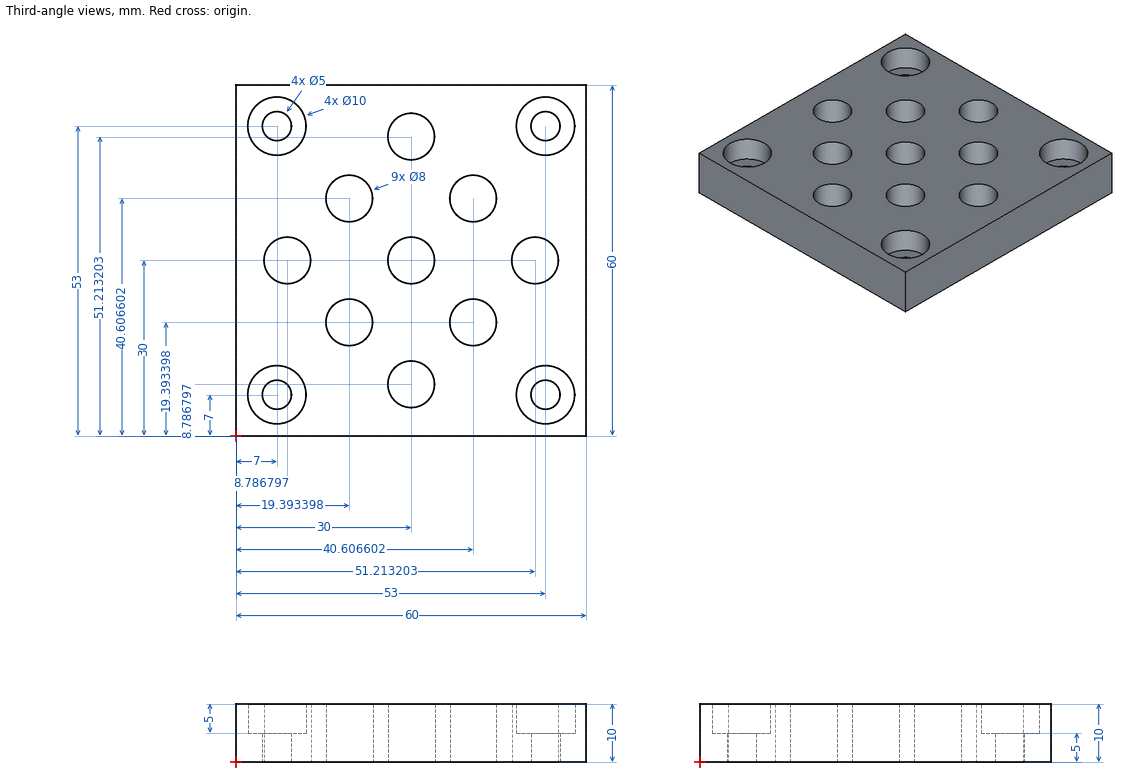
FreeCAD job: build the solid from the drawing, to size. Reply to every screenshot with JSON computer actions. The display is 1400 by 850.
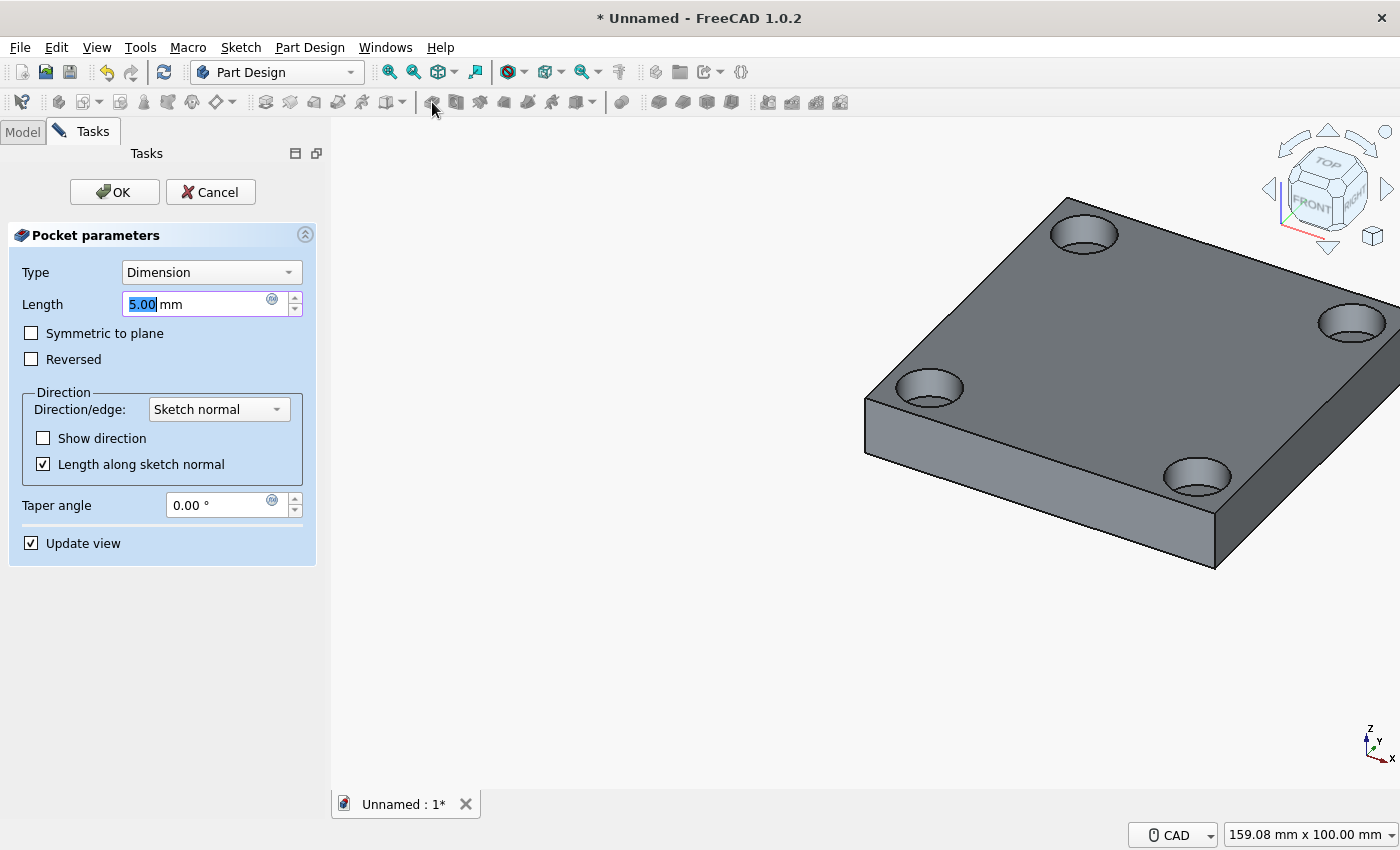
{"action": "type", "text": "5"}
{"action": "key", "text": "Tab"}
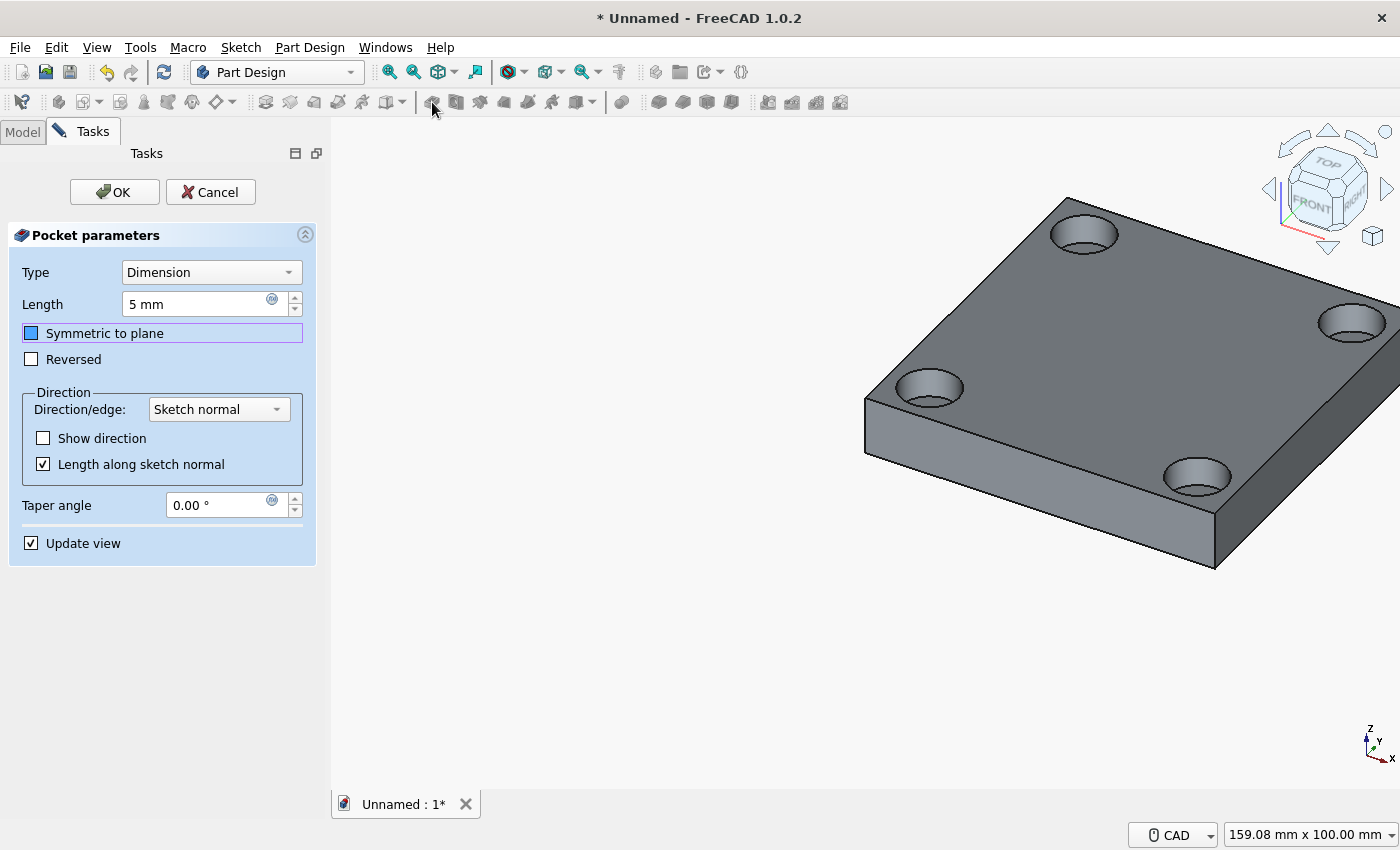
{"action": "left_click", "coordinate": [115, 192]}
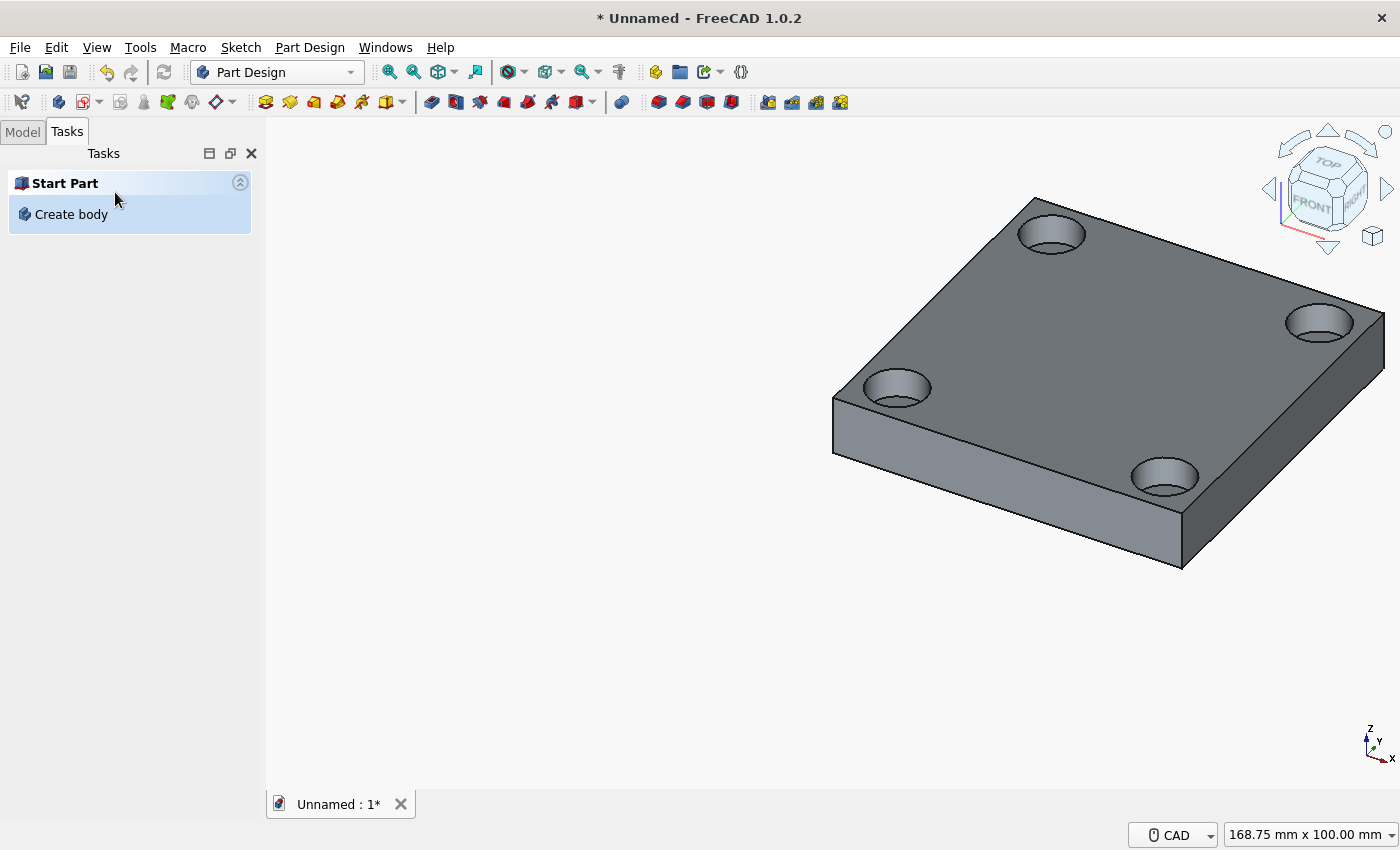
{"action": "key", "text": "0"}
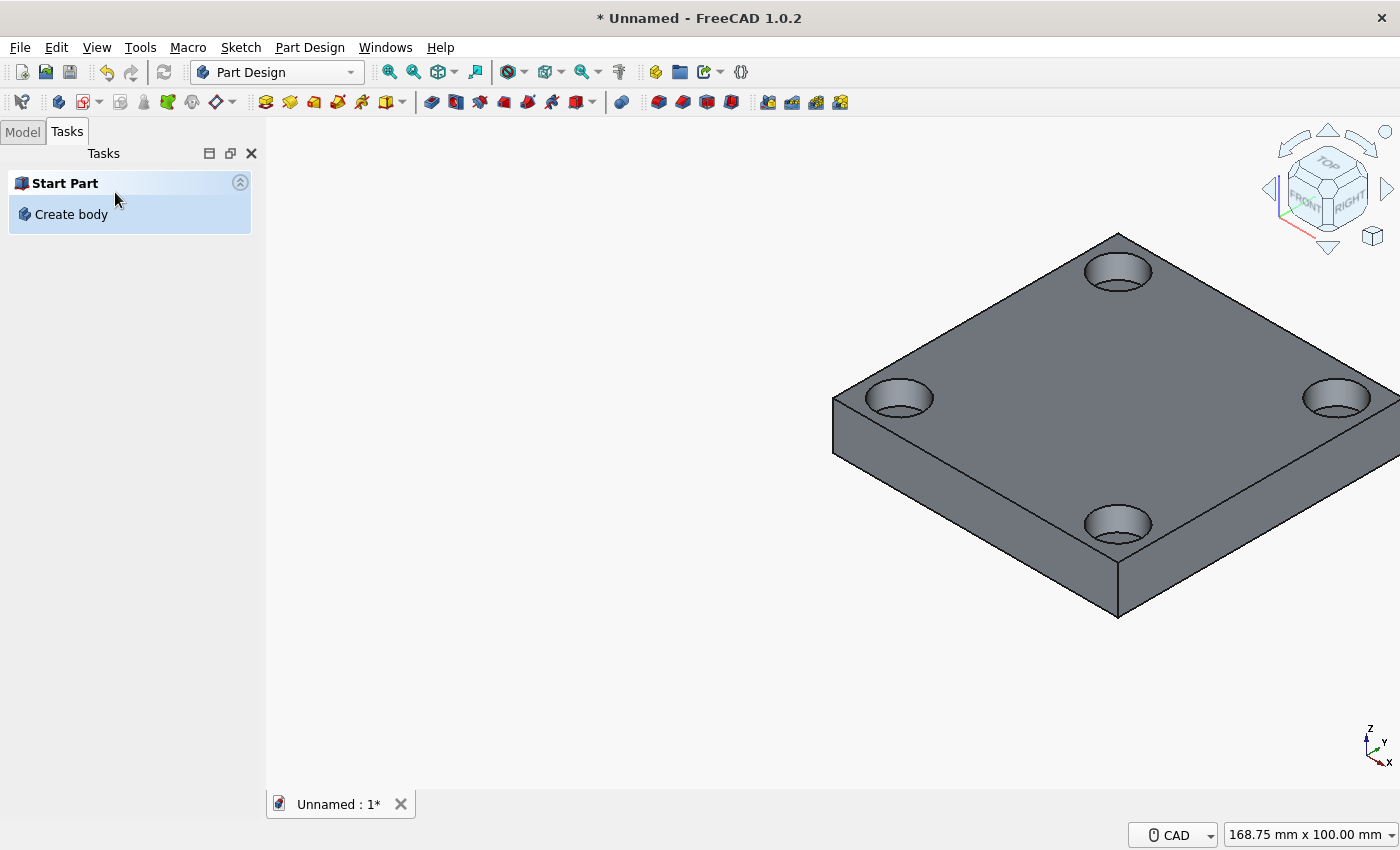
{"action": "left_click", "coordinate": [390, 72]}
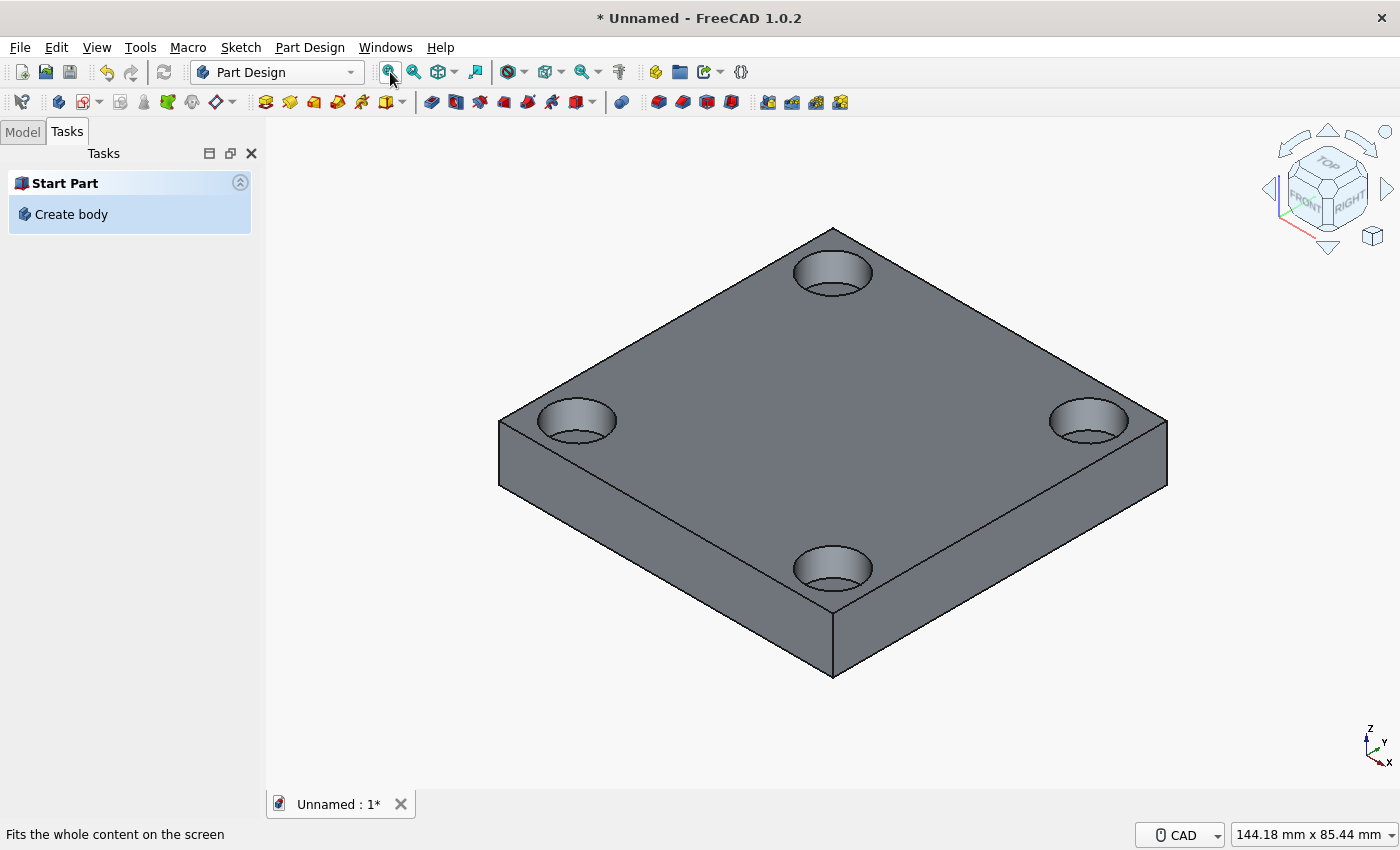
{"action": "key", "text": "2"}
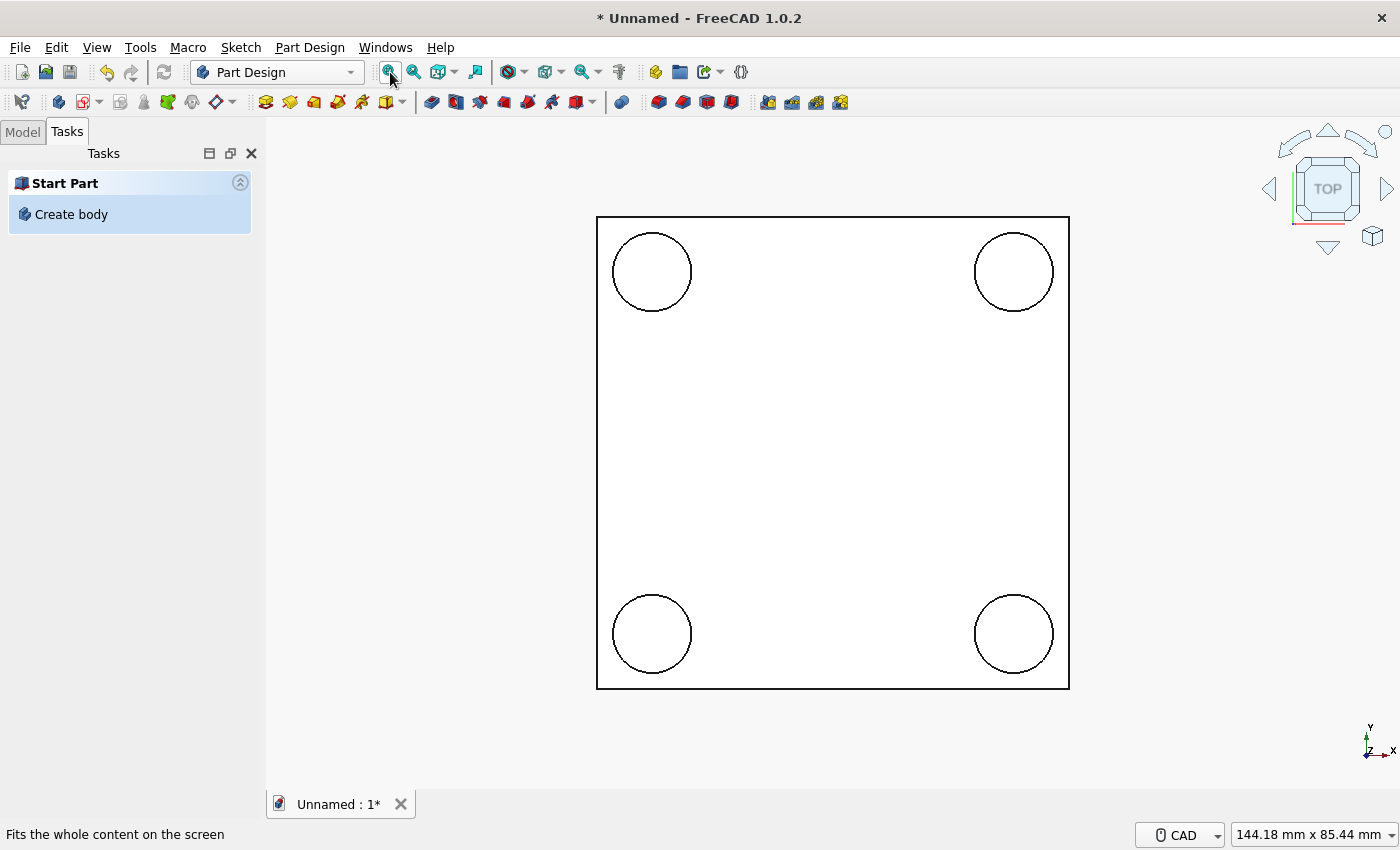
{"action": "left_click", "coordinate": [1014, 271]}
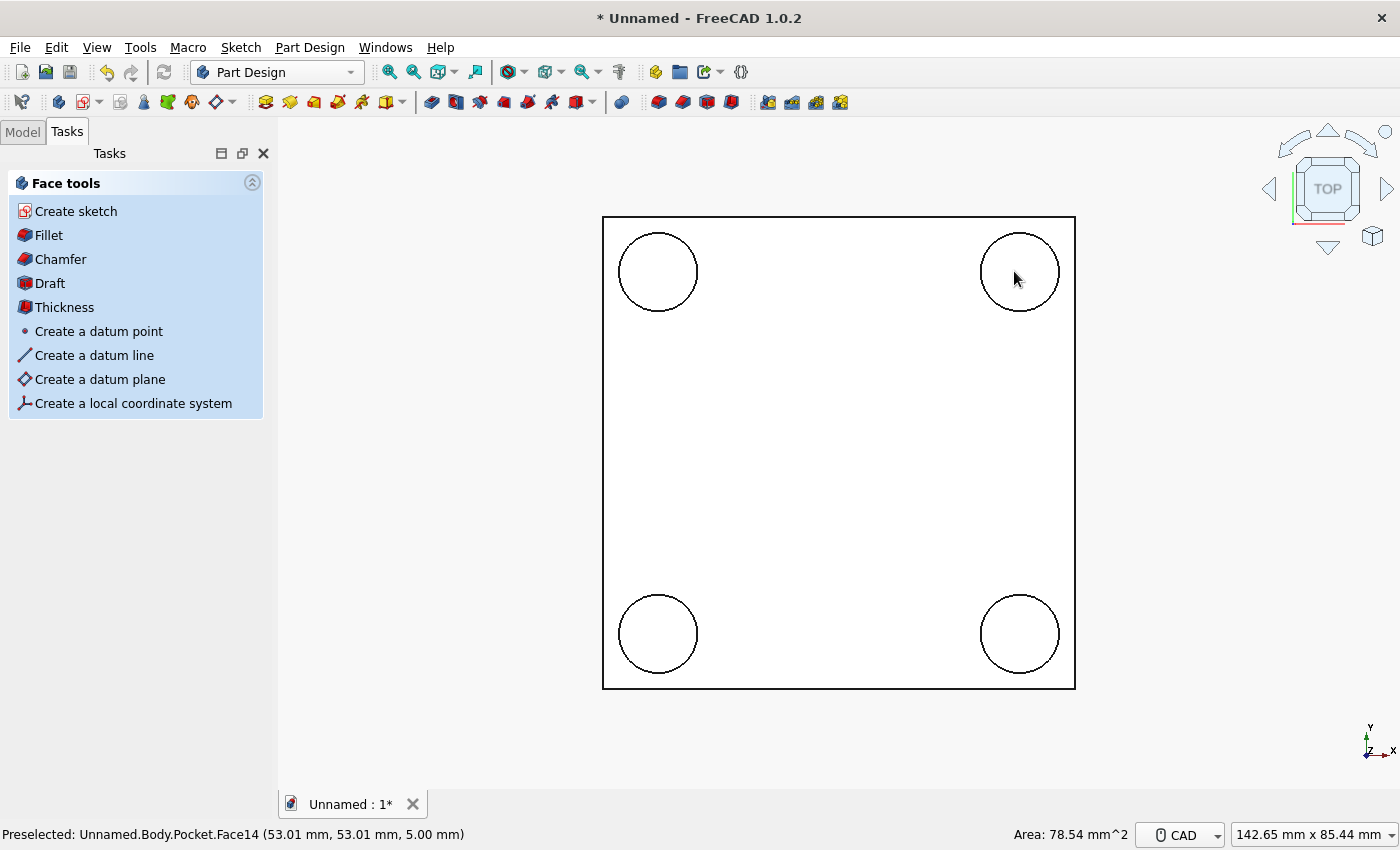
{"action": "left_click", "coordinate": [84, 102]}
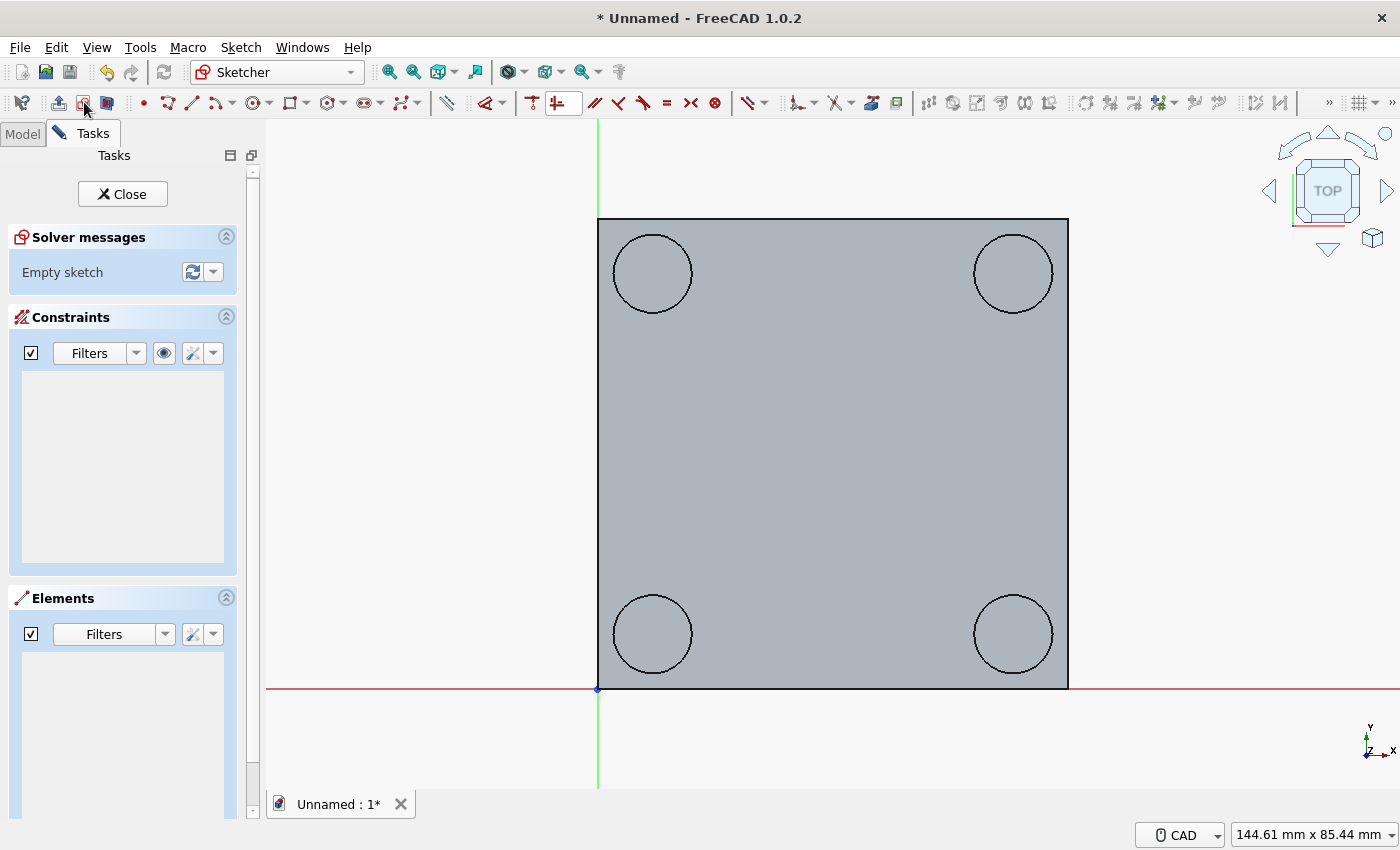
{"action": "left_click", "coordinate": [108, 104]}